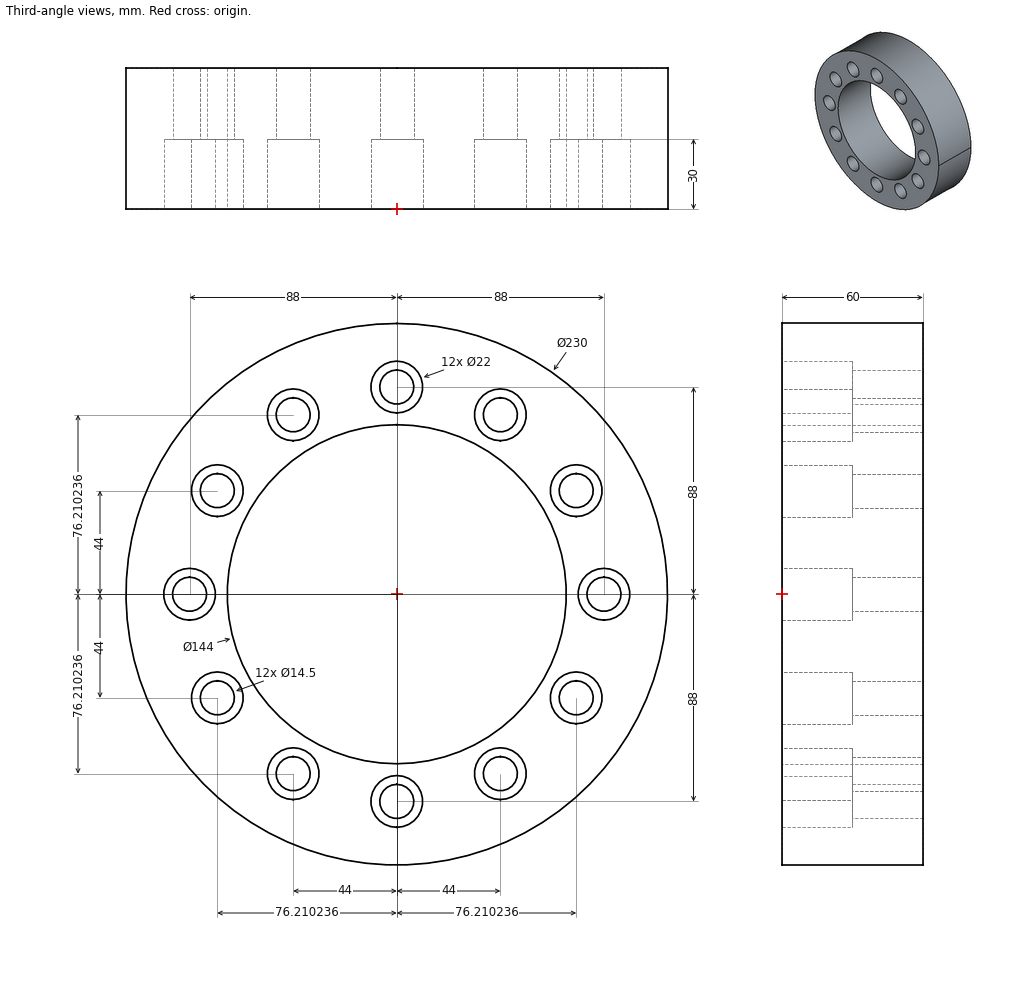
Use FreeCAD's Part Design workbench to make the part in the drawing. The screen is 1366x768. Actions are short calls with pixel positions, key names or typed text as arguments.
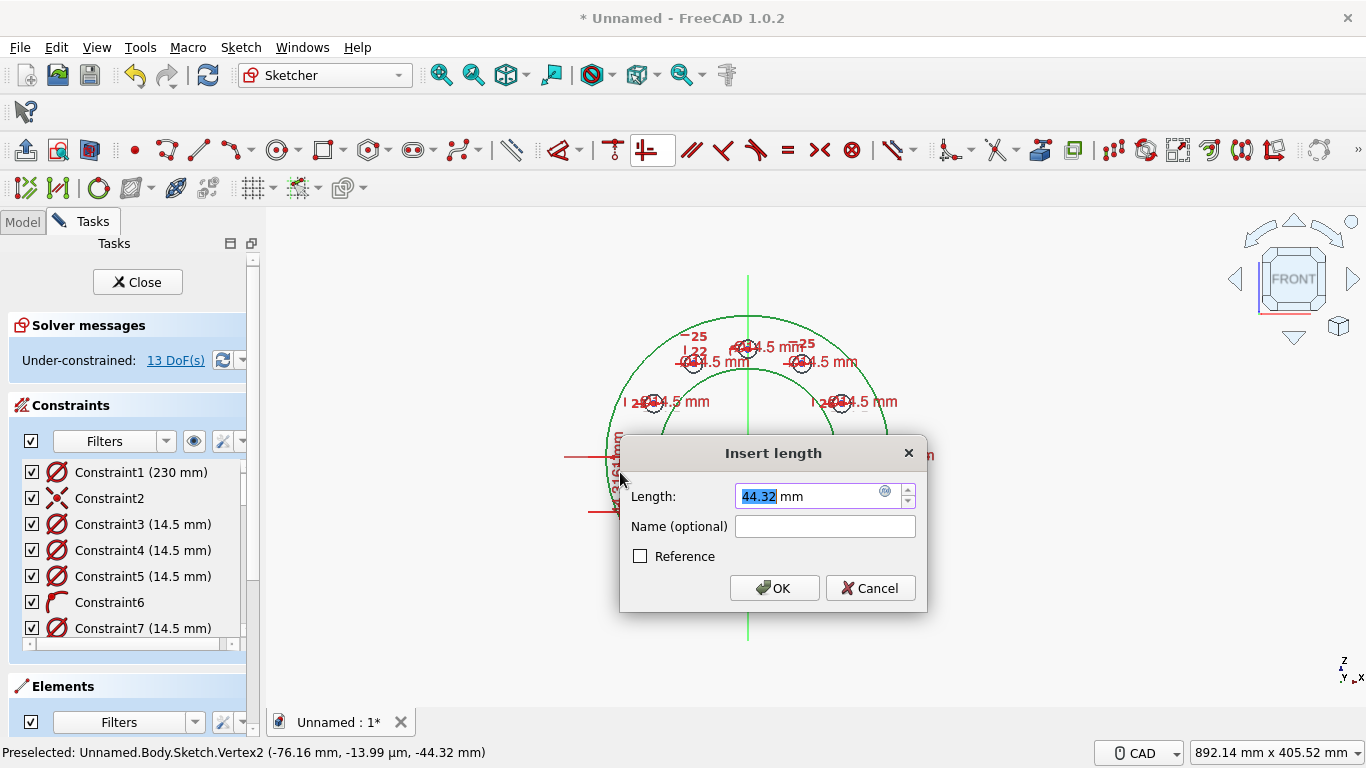
text(44)
key(Return)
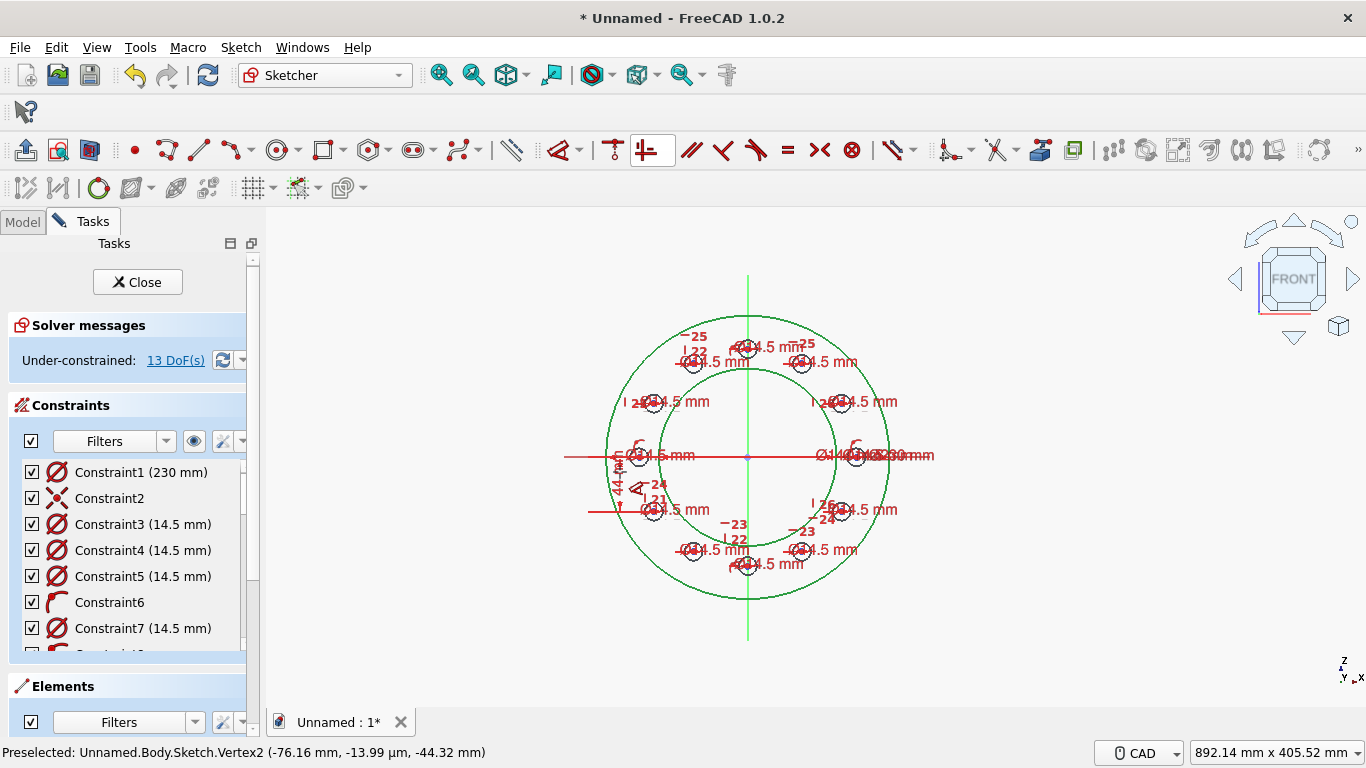
click(694, 552)
click(721, 423)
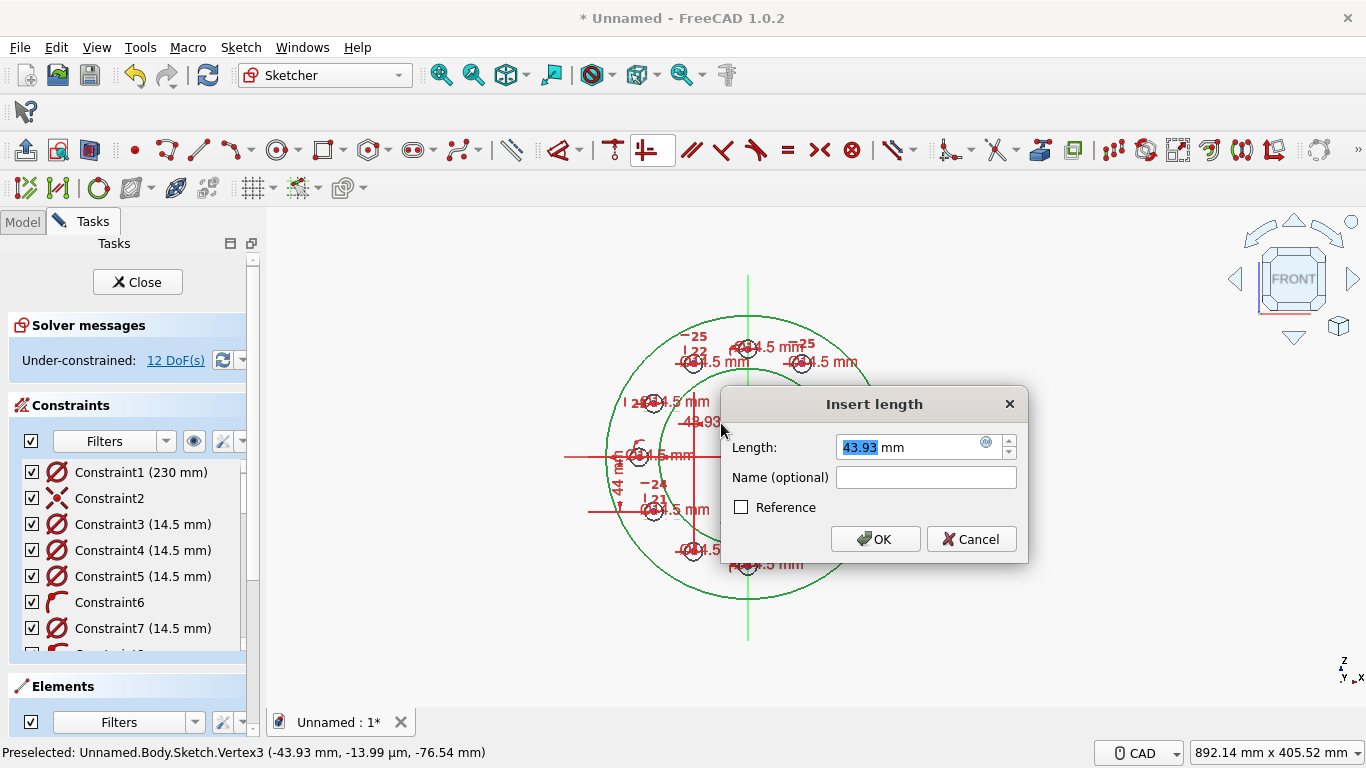
text(44)
key(Return)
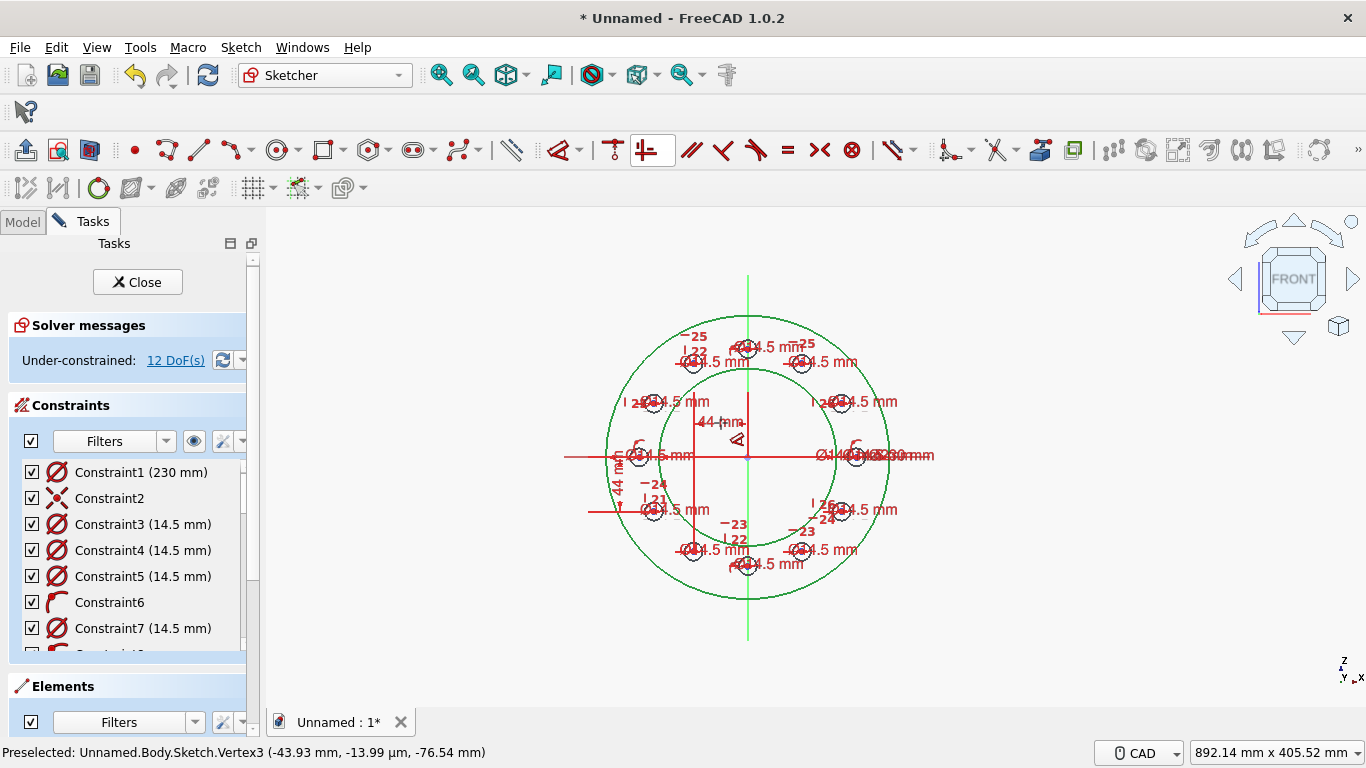
click(748, 566)
click(782, 512)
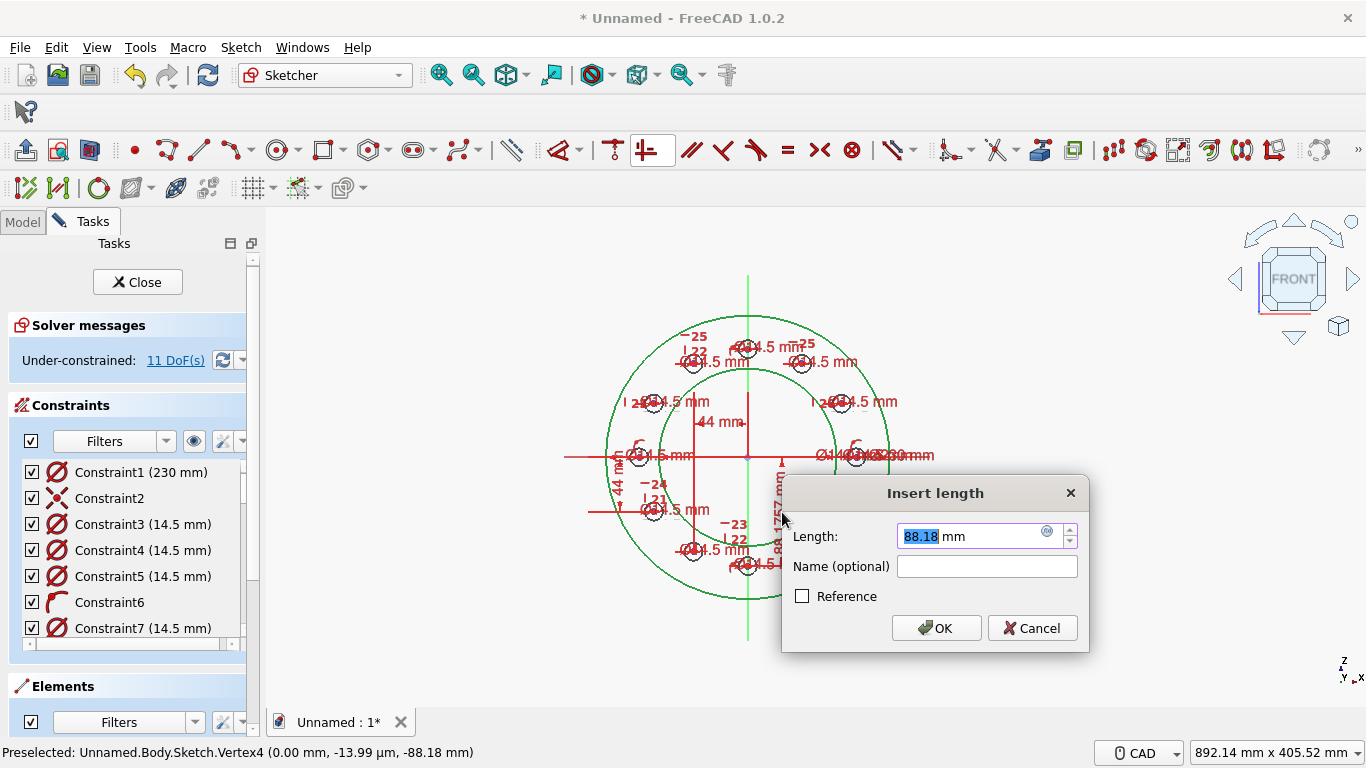
text(88)
key(Return)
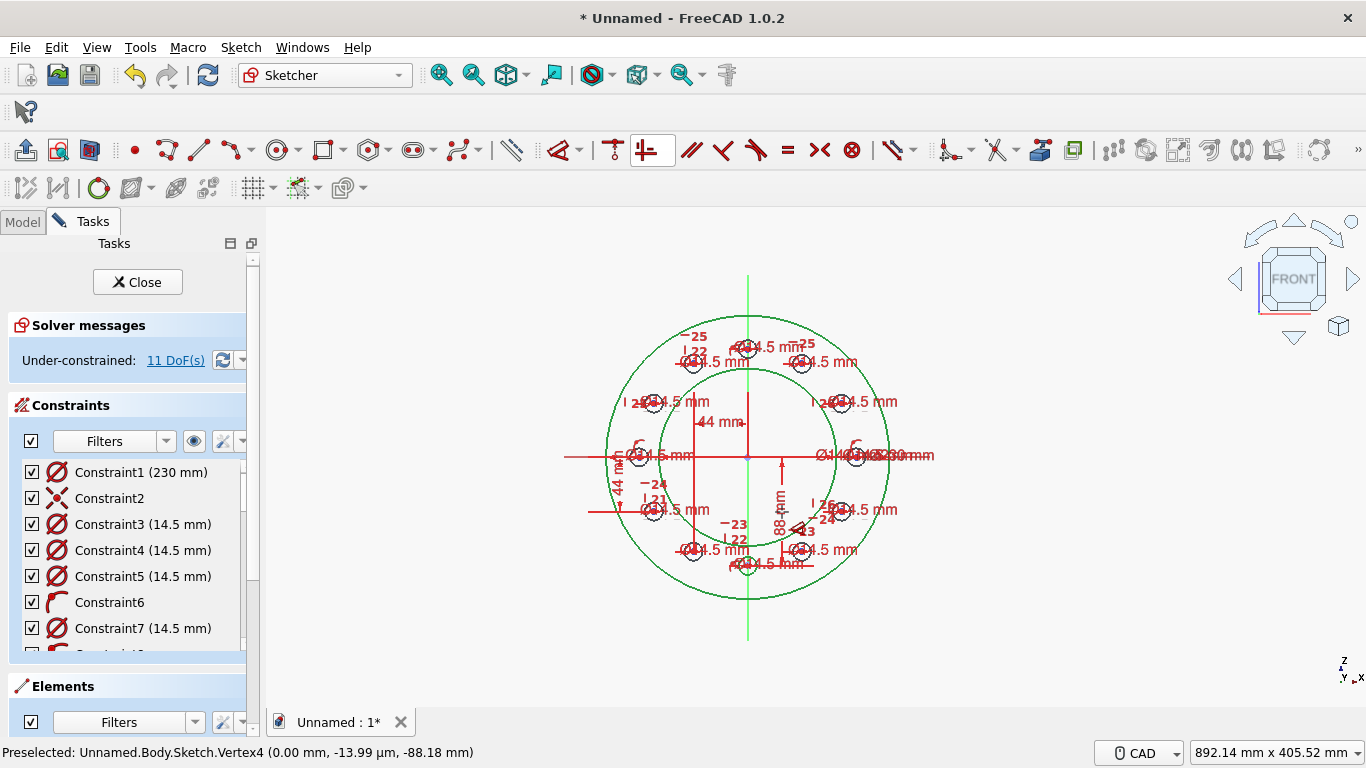
click(639, 457)
click(693, 491)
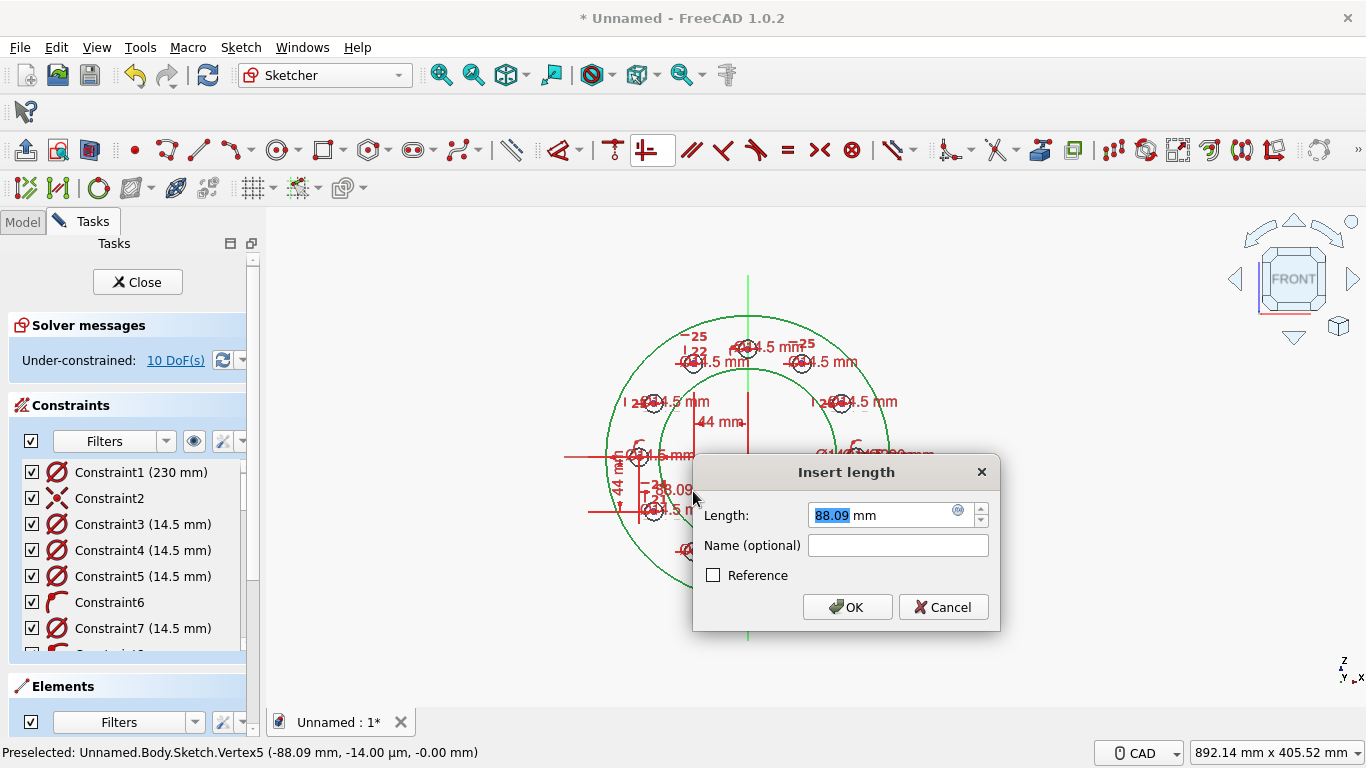
text(88)
key(Return)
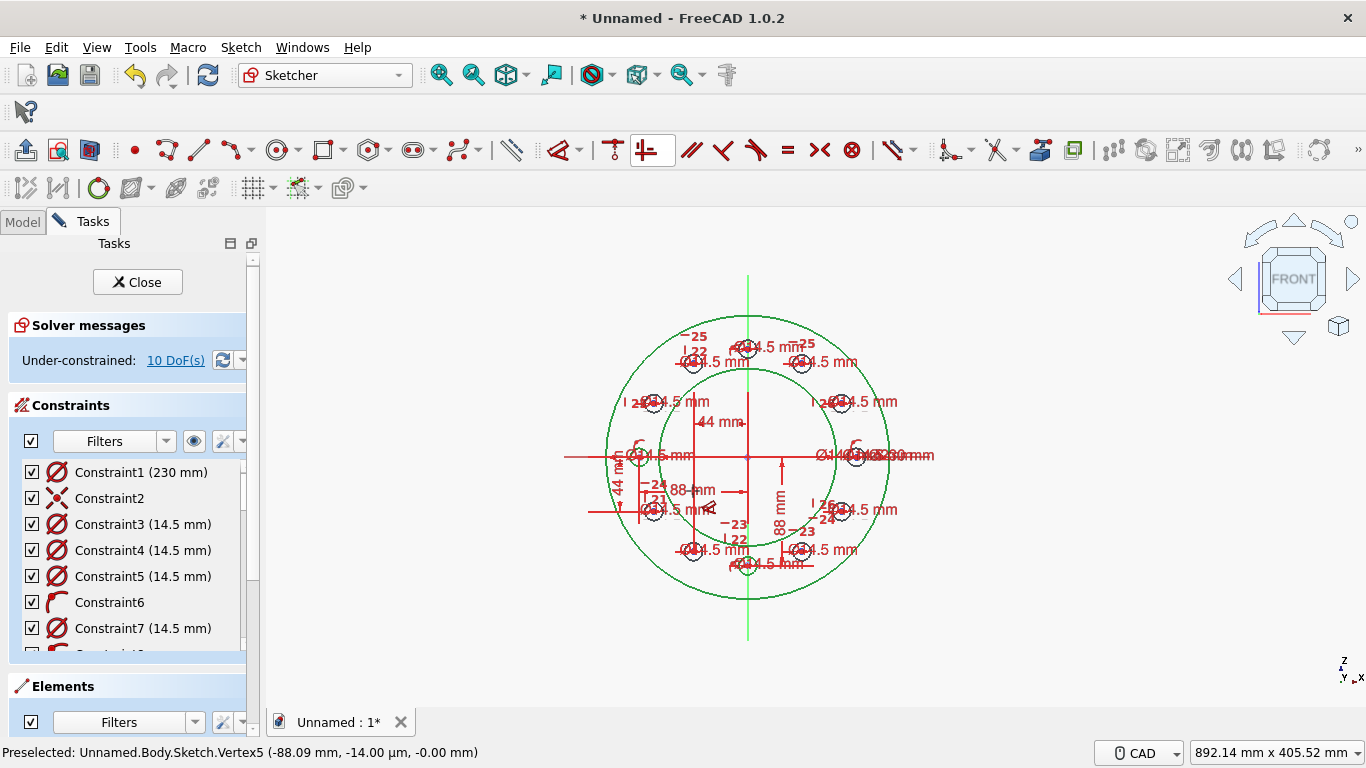
click(654, 404)
click(620, 443)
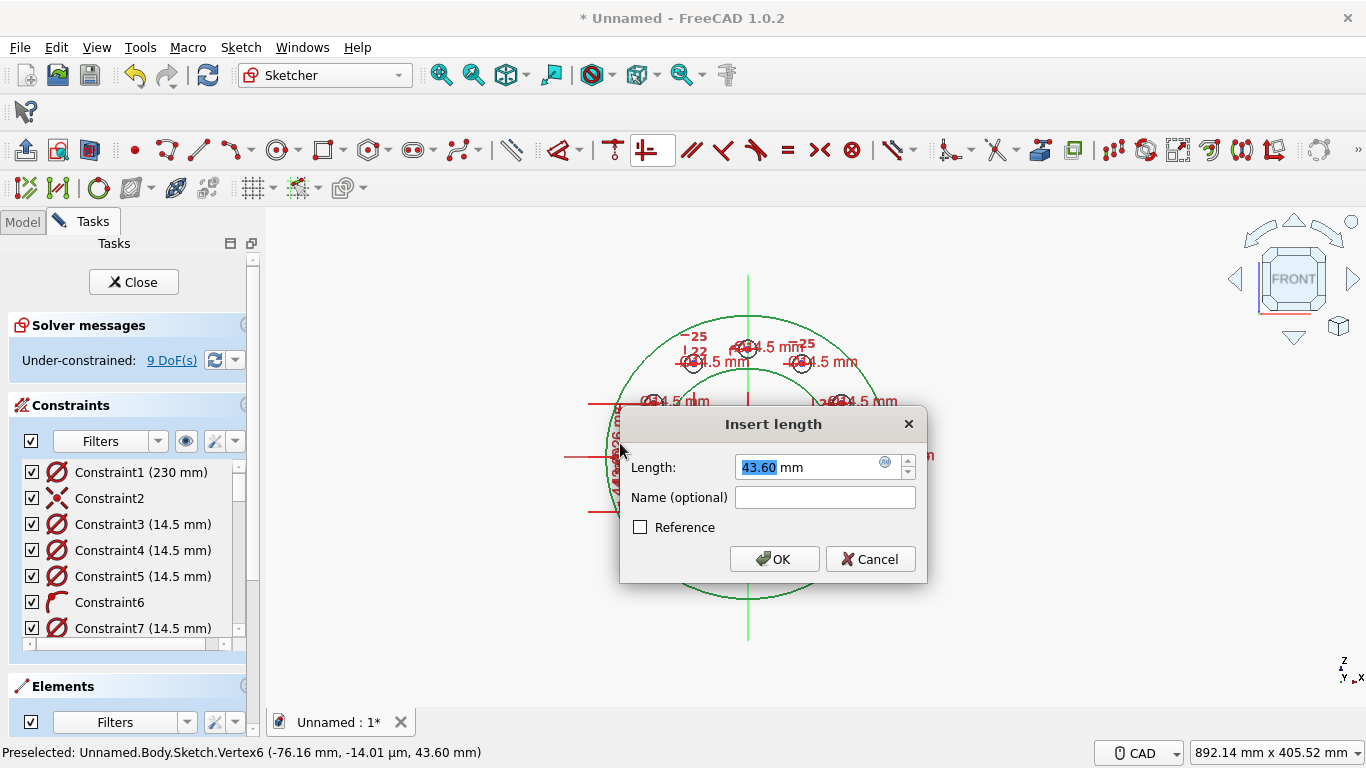
text(44)
key(Return)